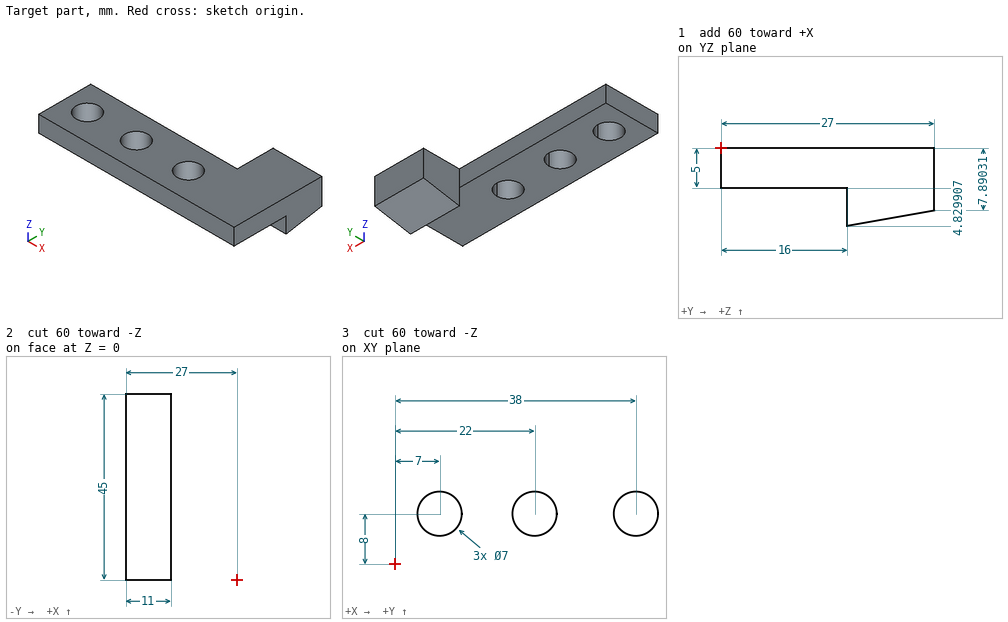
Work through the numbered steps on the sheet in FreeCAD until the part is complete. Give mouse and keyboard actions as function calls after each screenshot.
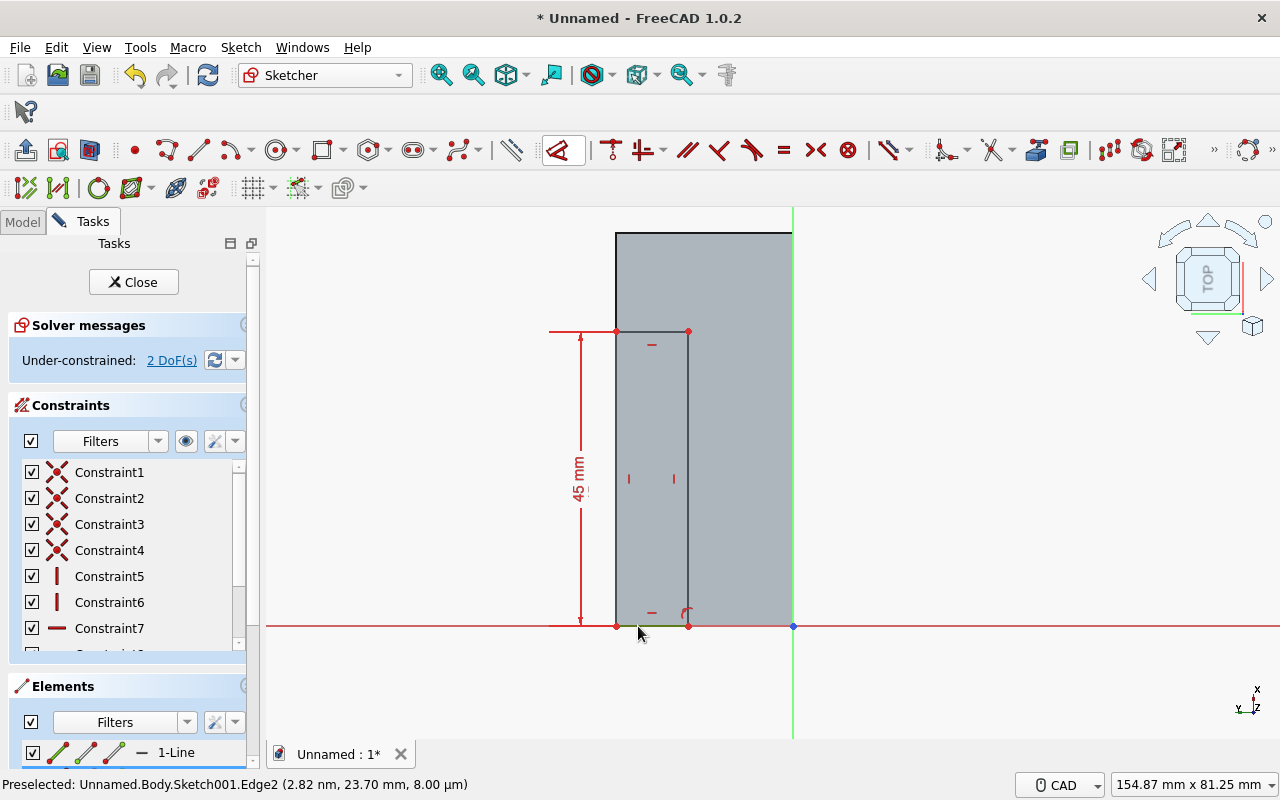
click(580, 150)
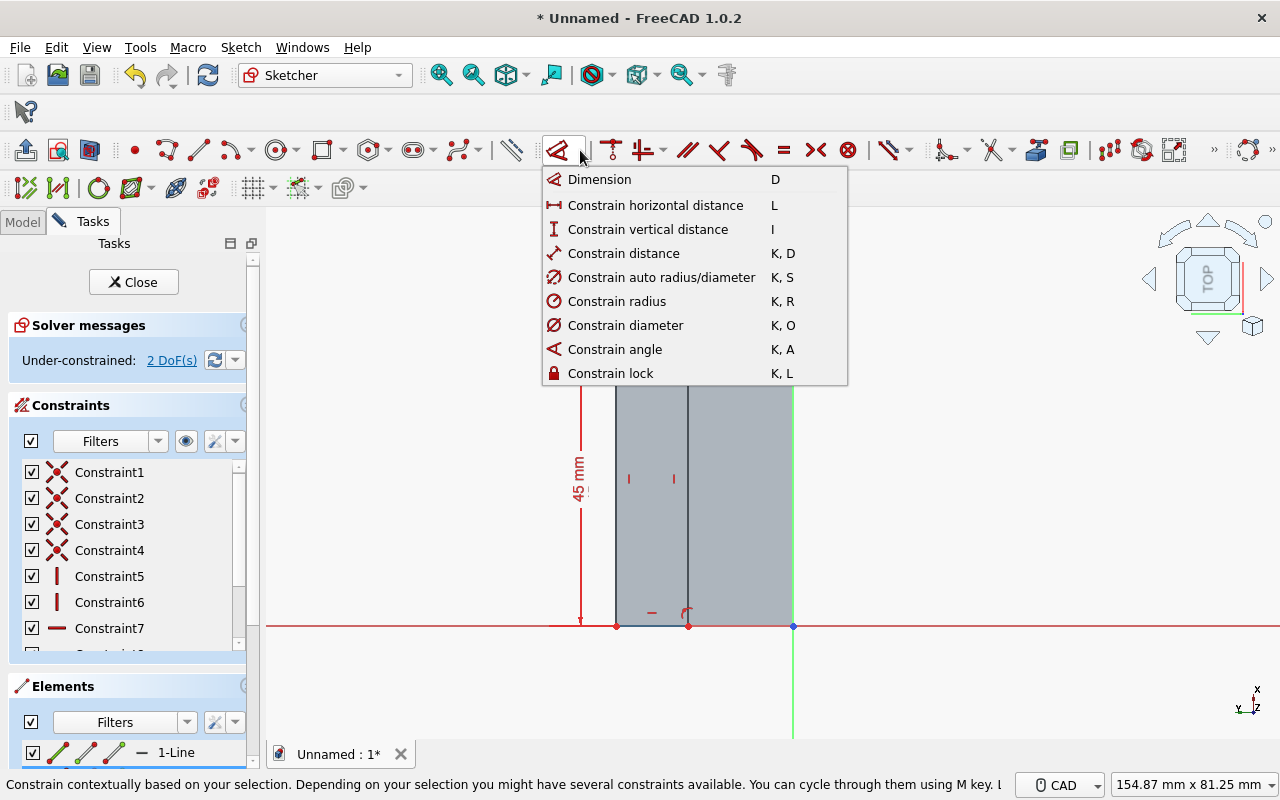
click(695, 205)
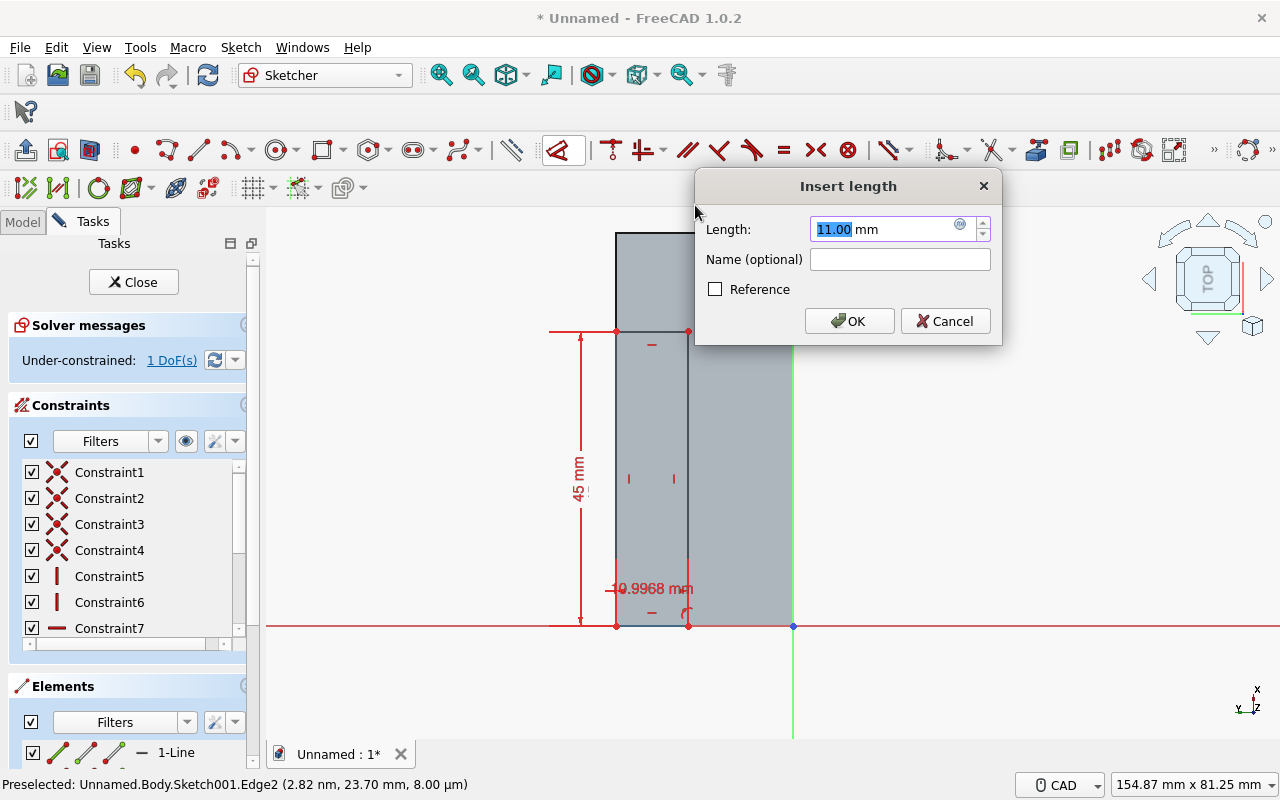
text(11)
key(Return)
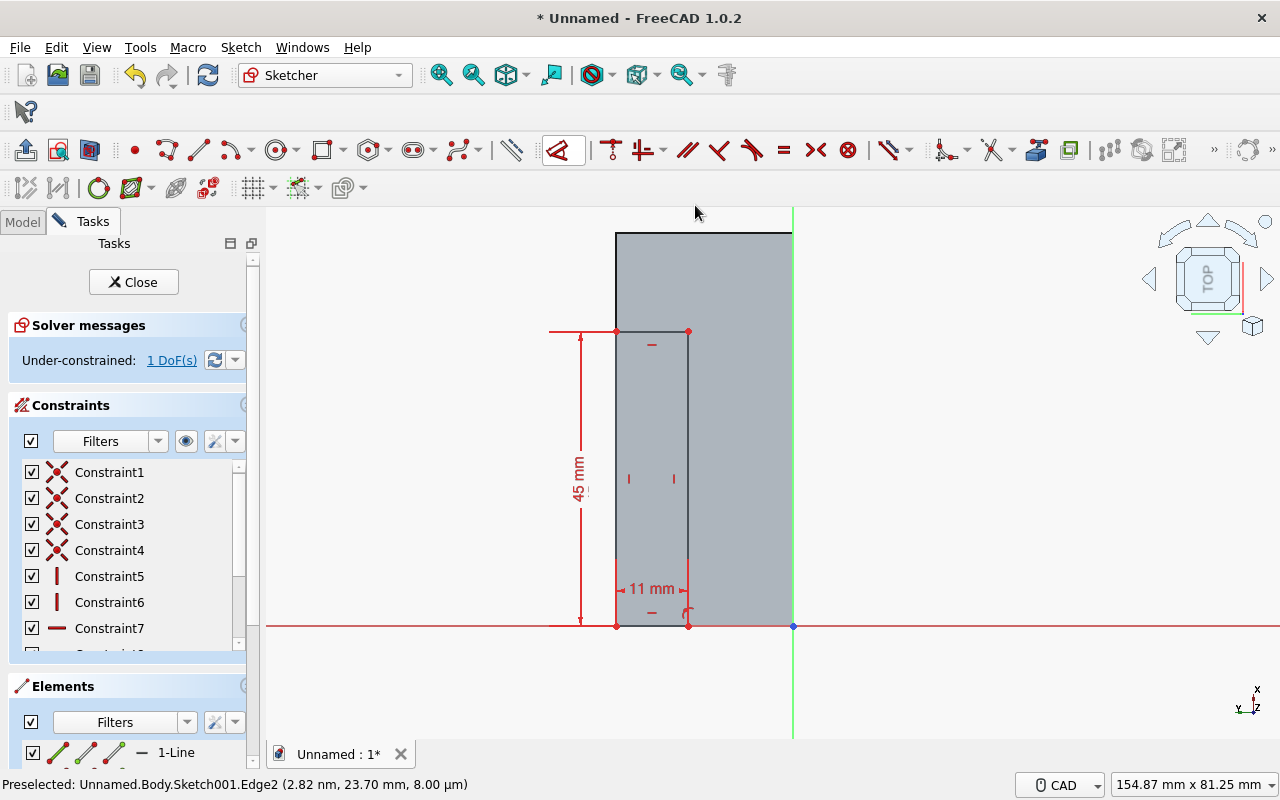
click(616, 332)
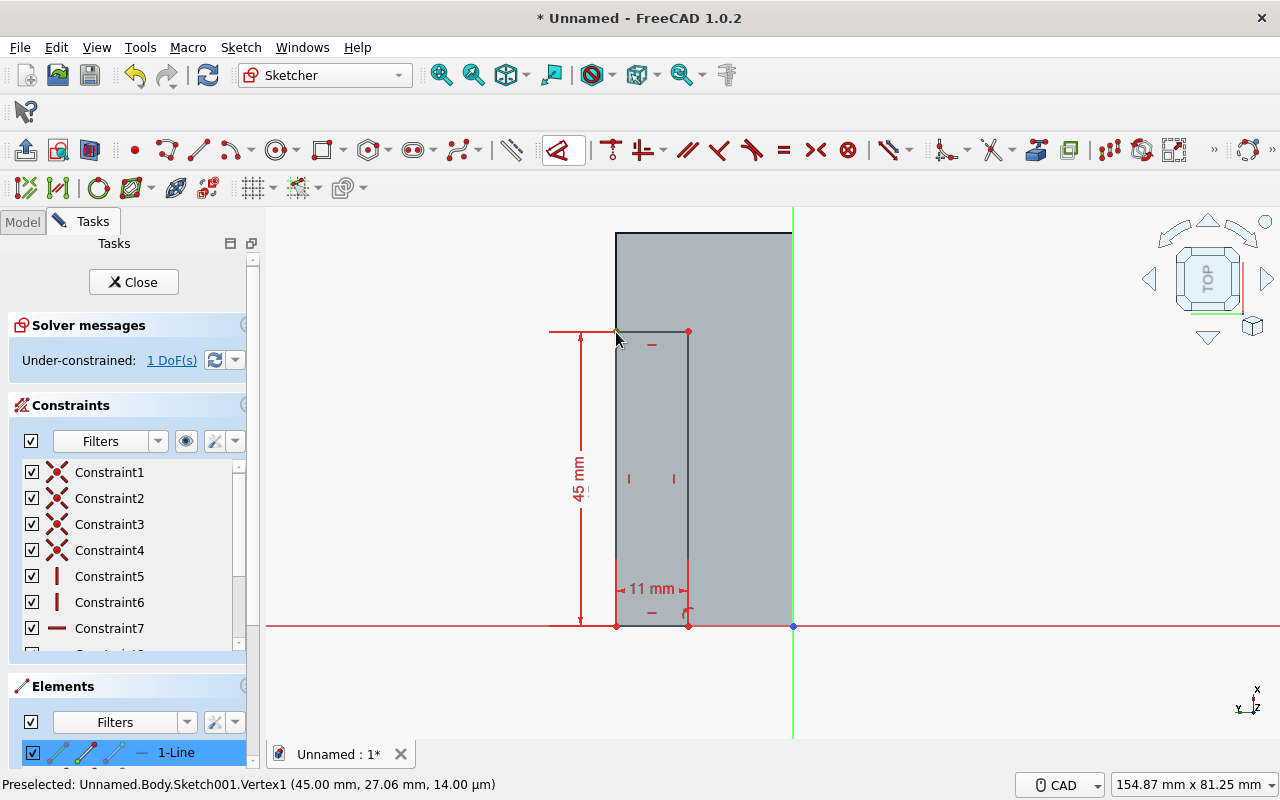
click(580, 150)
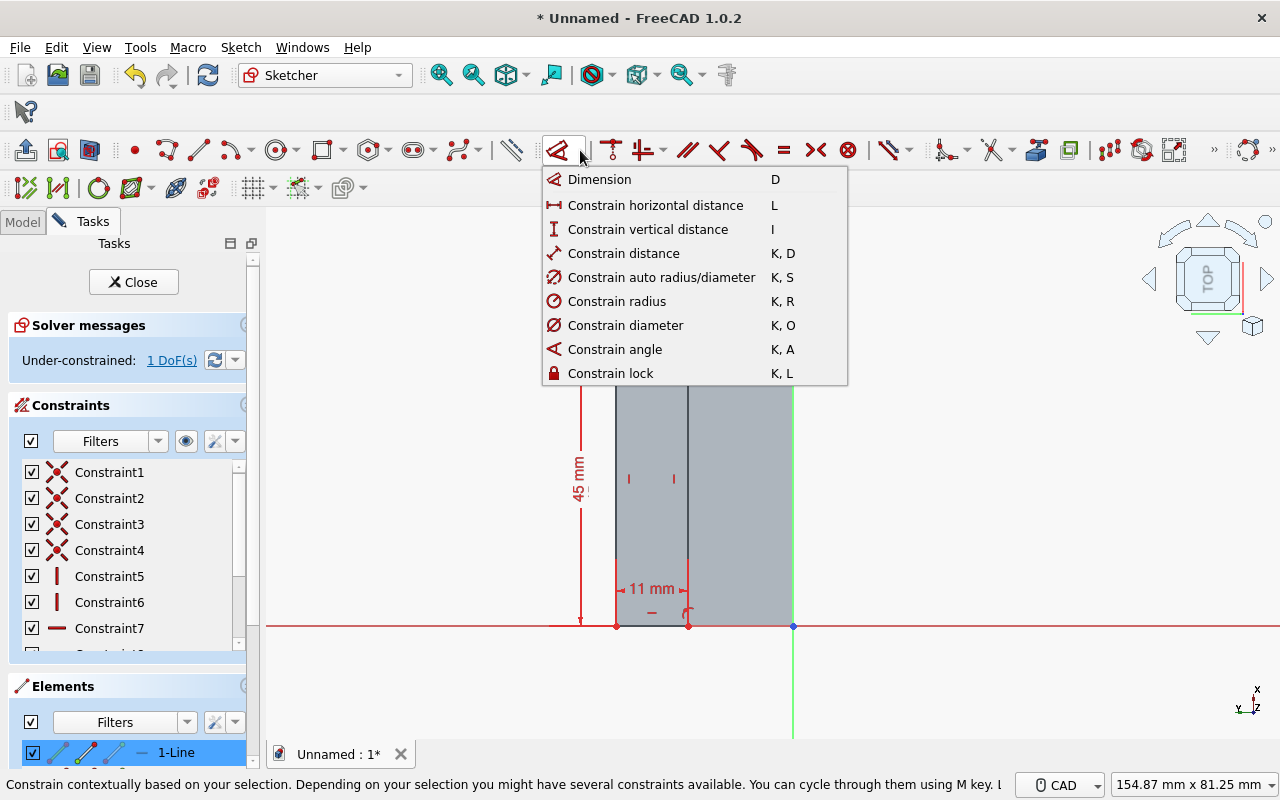
click(695, 205)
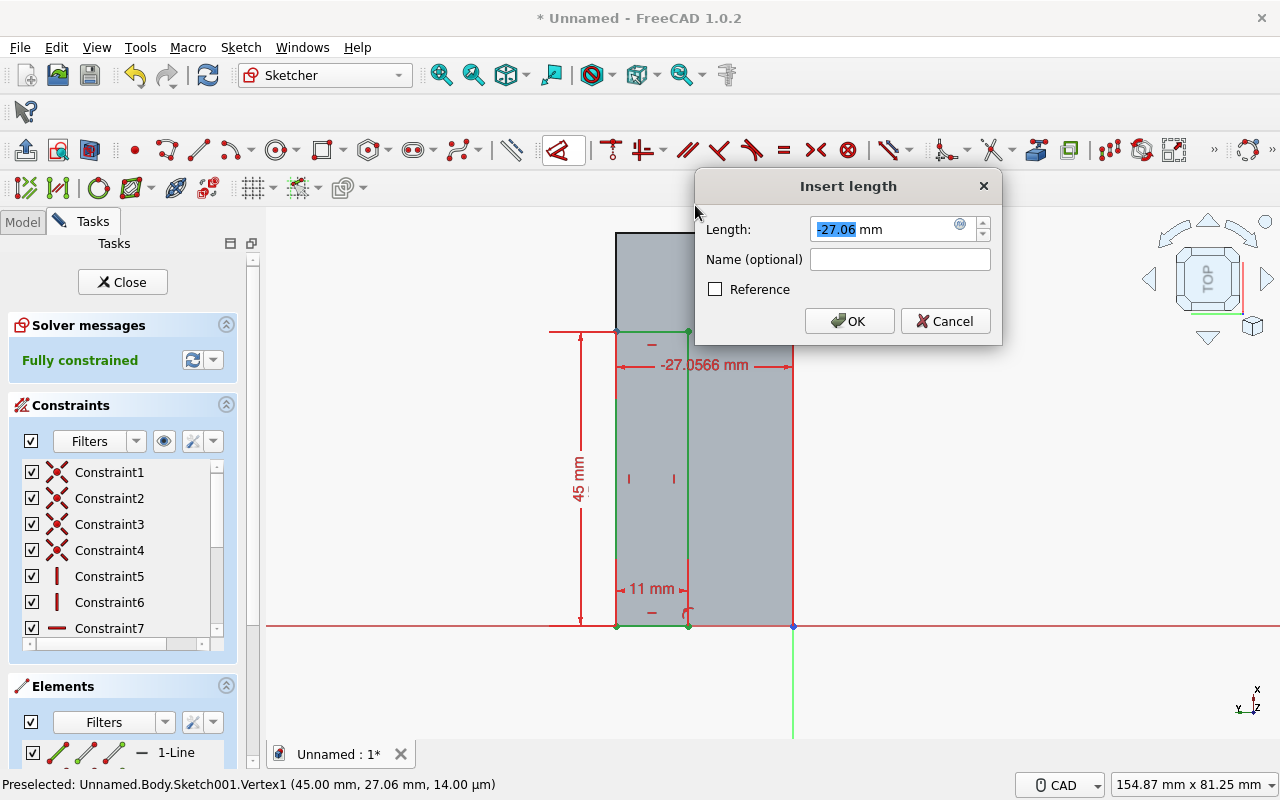
text(-27)
key(Return)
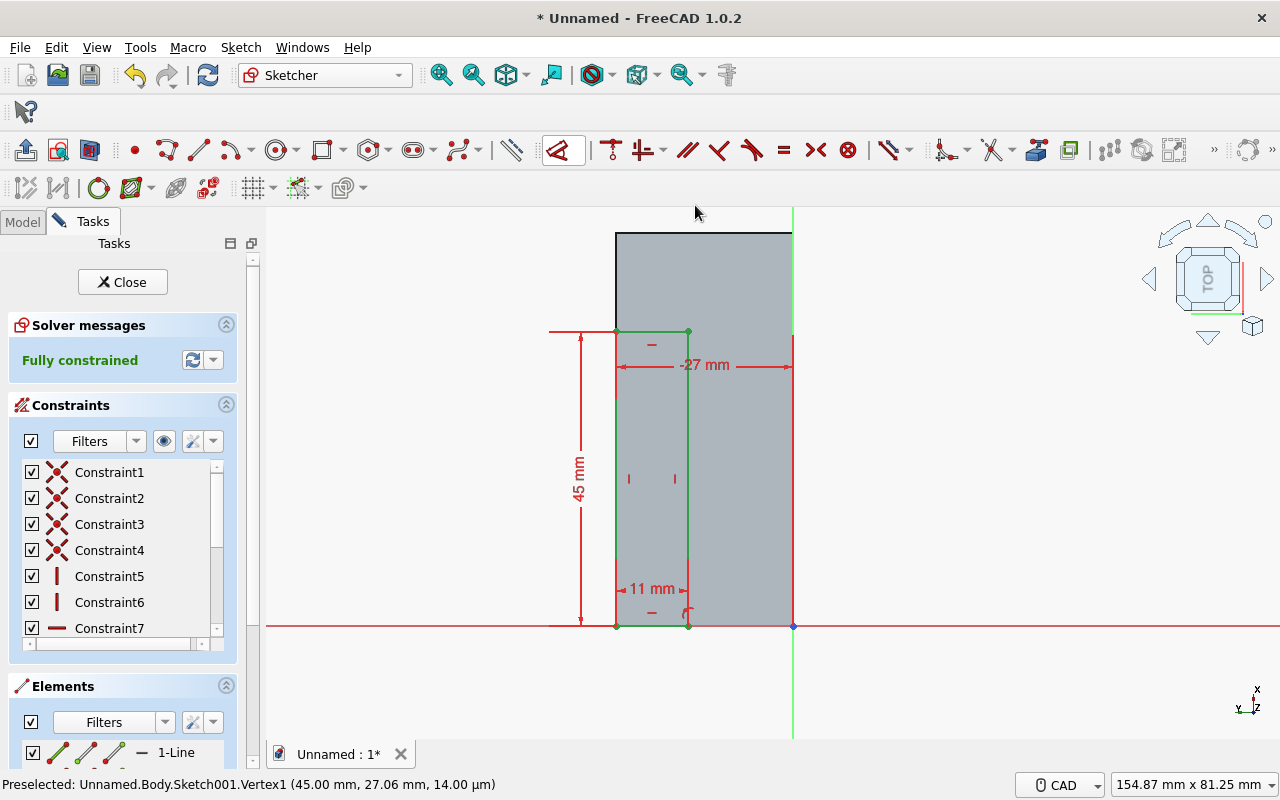
click(123, 282)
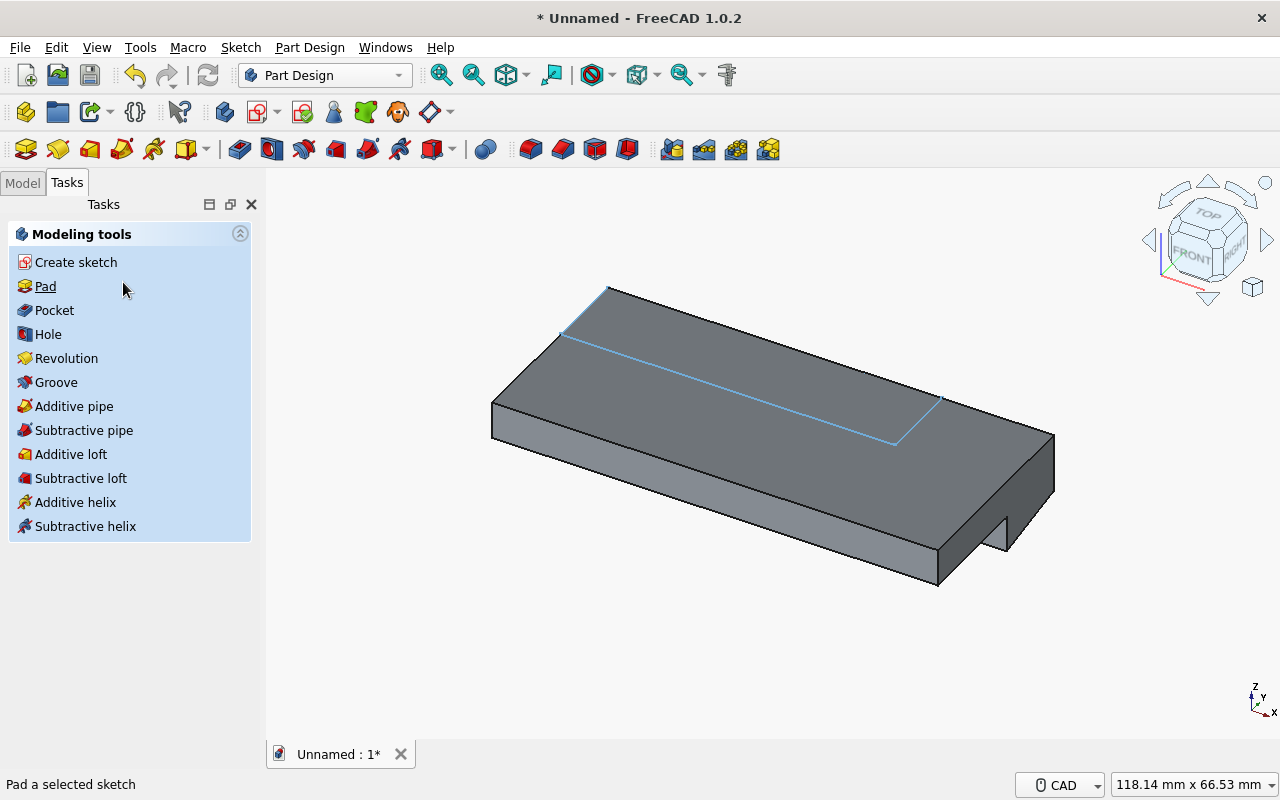
click(240, 150)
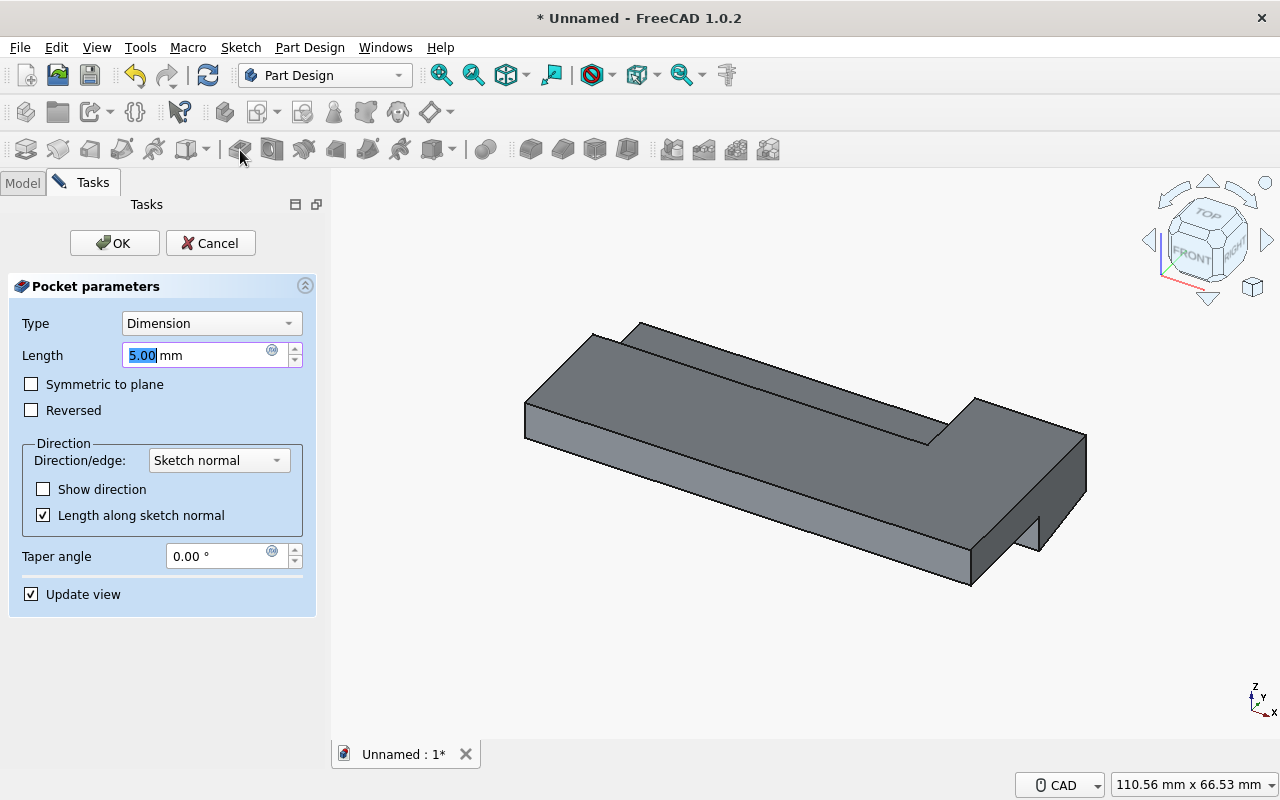
text(60)
key(Tab)